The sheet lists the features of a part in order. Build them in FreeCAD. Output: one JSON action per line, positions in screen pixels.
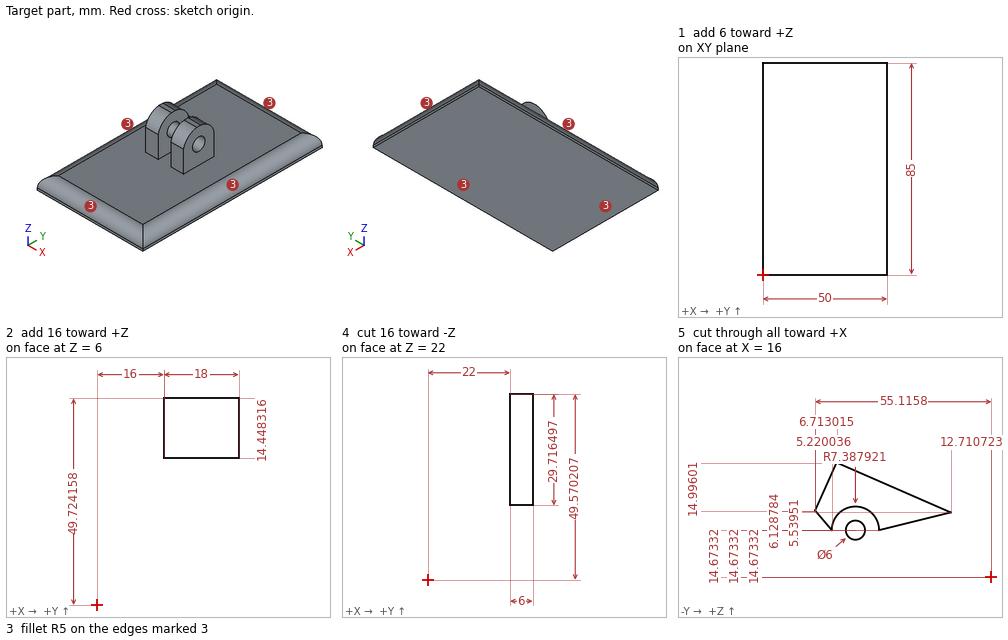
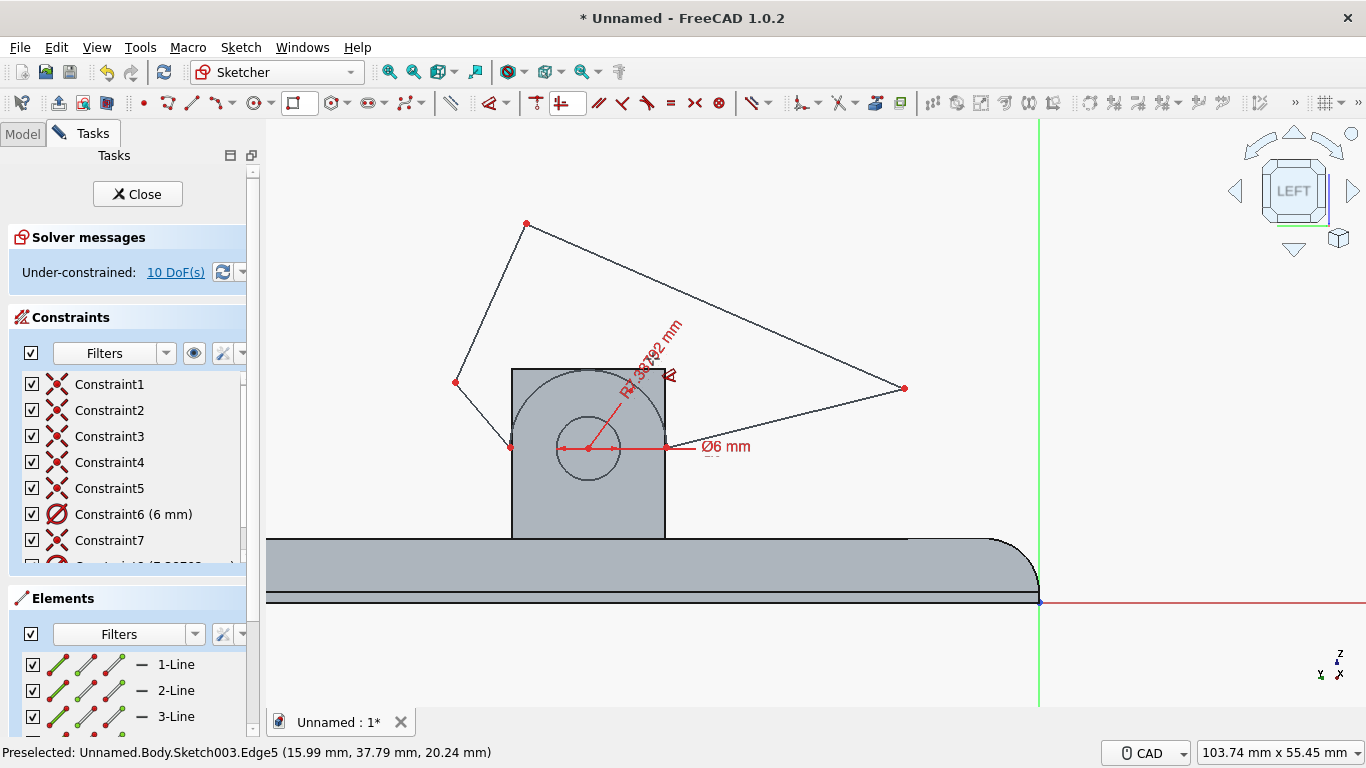
{"action": "left_click", "coordinate": [455, 383]}
{"action": "left_click", "coordinate": [747, 637]}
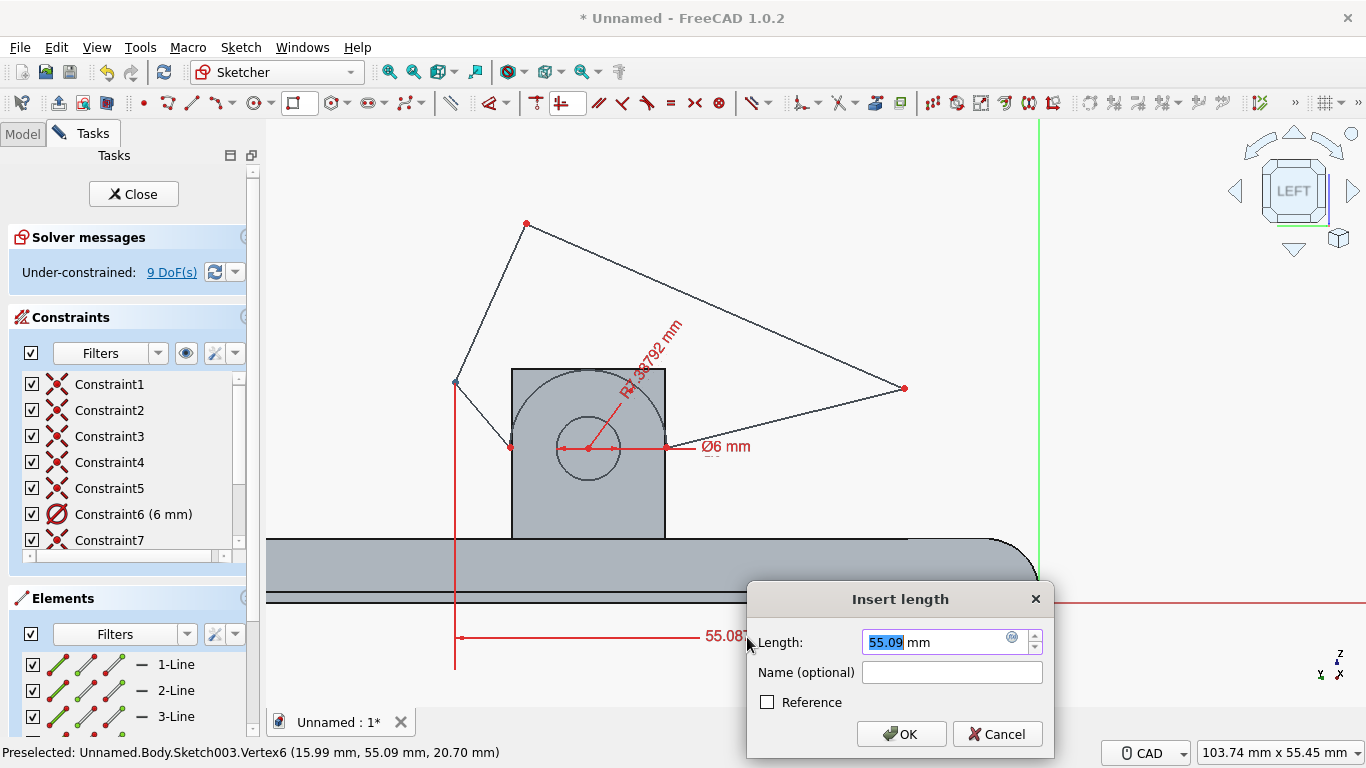
{"action": "type", "text": "55.1158"}
{"action": "key", "text": "Return"}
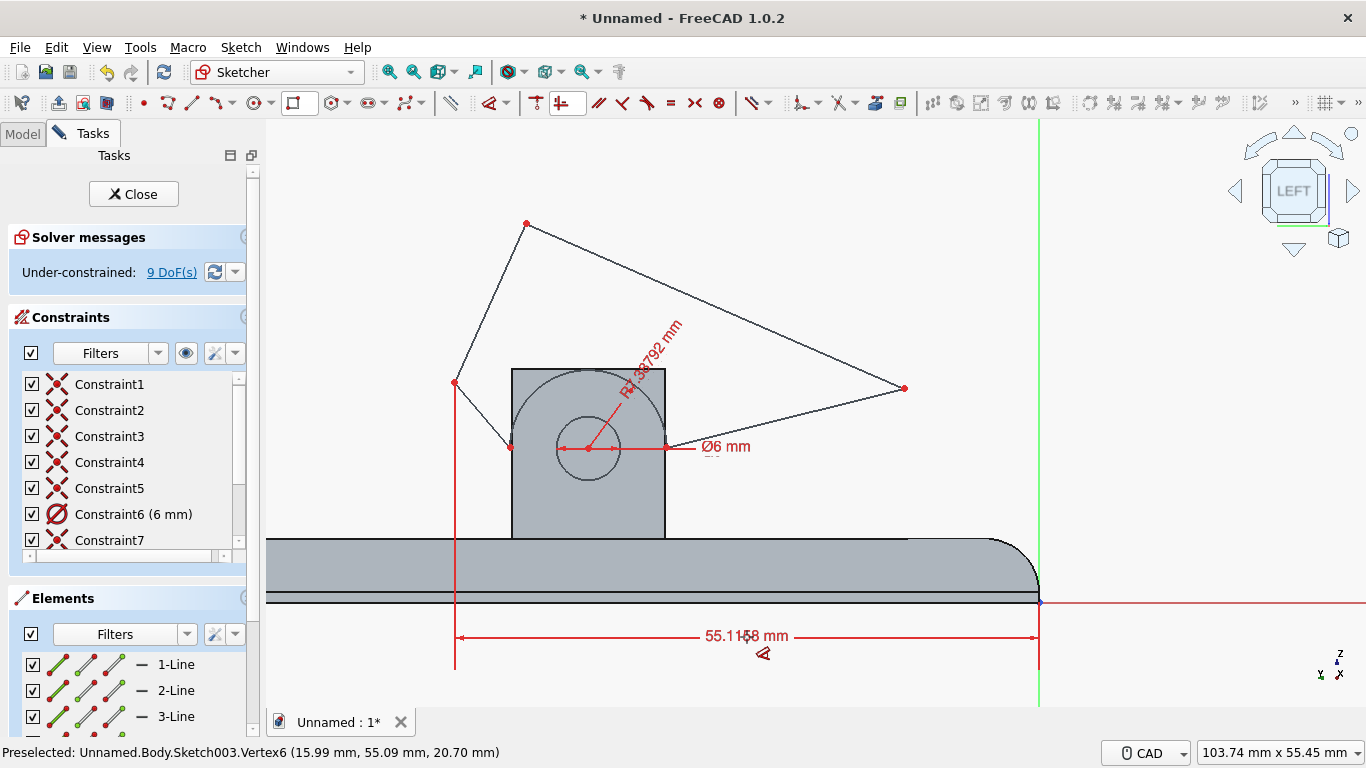
{"action": "left_click", "coordinate": [738, 430]}
{"action": "left_click", "coordinate": [938, 419]}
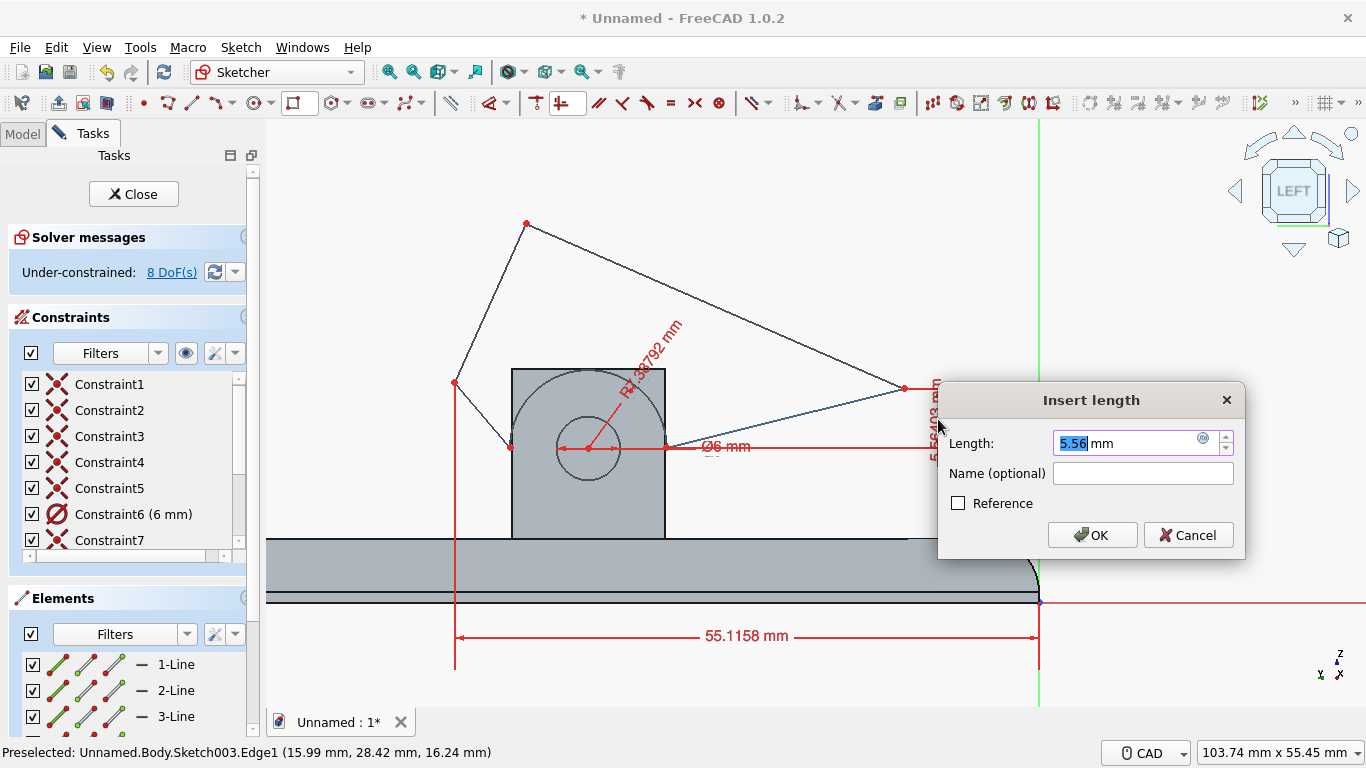
{"action": "type", "text": "5.53951"}
{"action": "key", "text": "Return"}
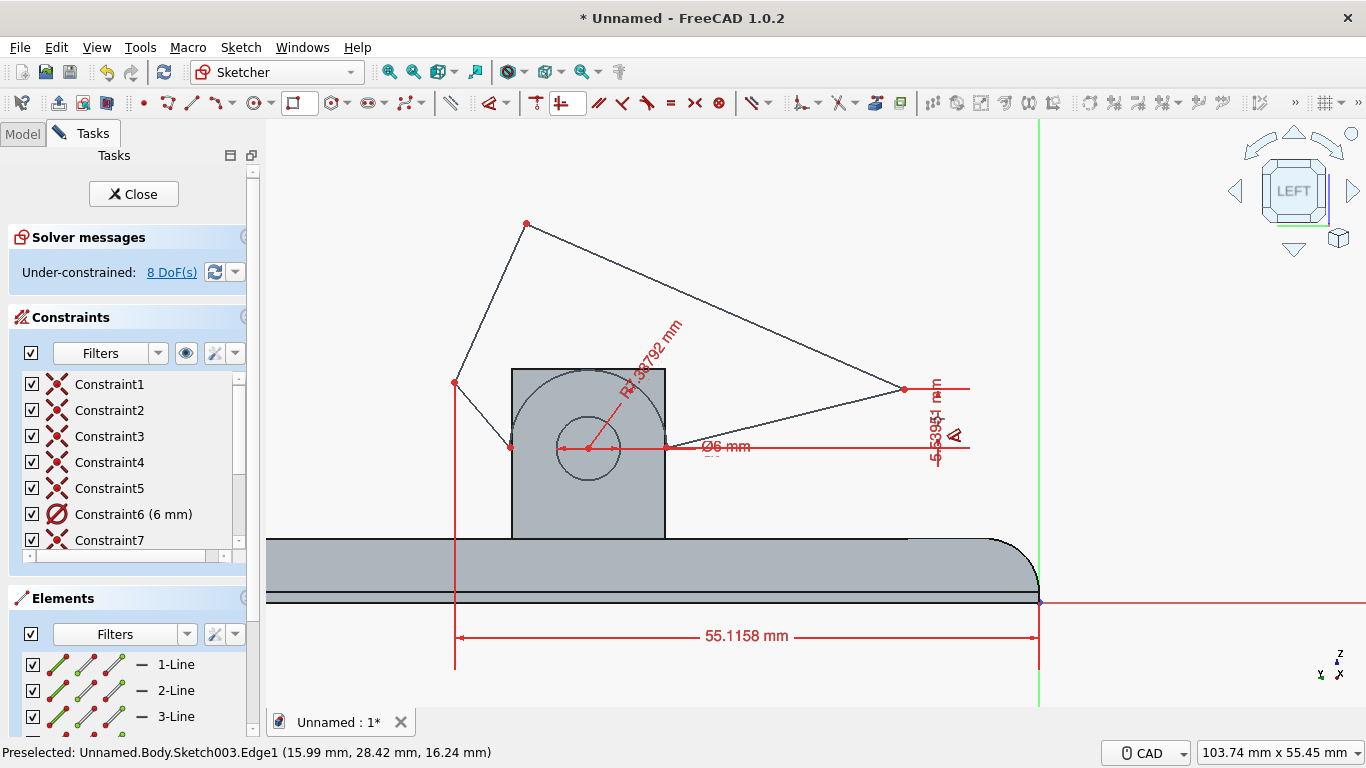
{"action": "left_click", "coordinate": [588, 449]}
{"action": "left_click", "coordinate": [1073, 526]}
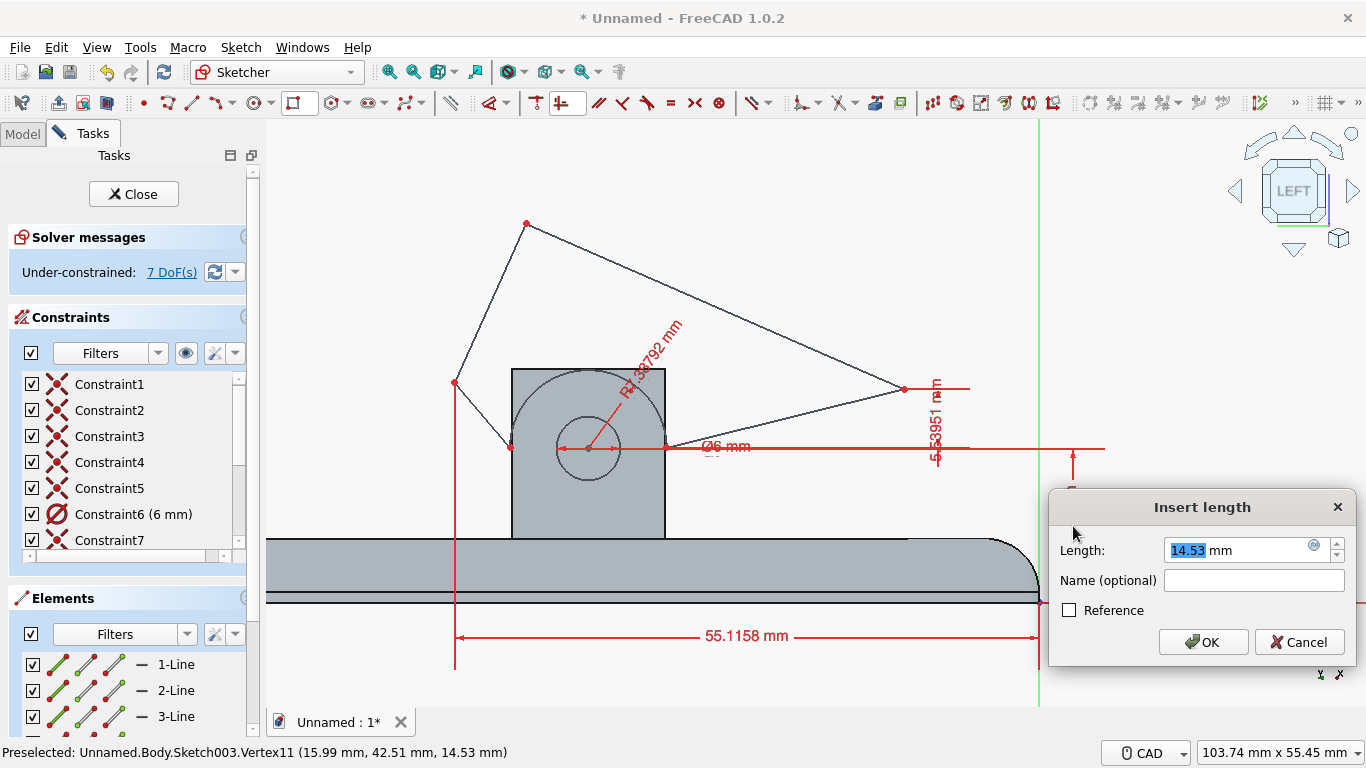
{"action": "type", "text": "14.67332"}
{"action": "key", "text": "Return"}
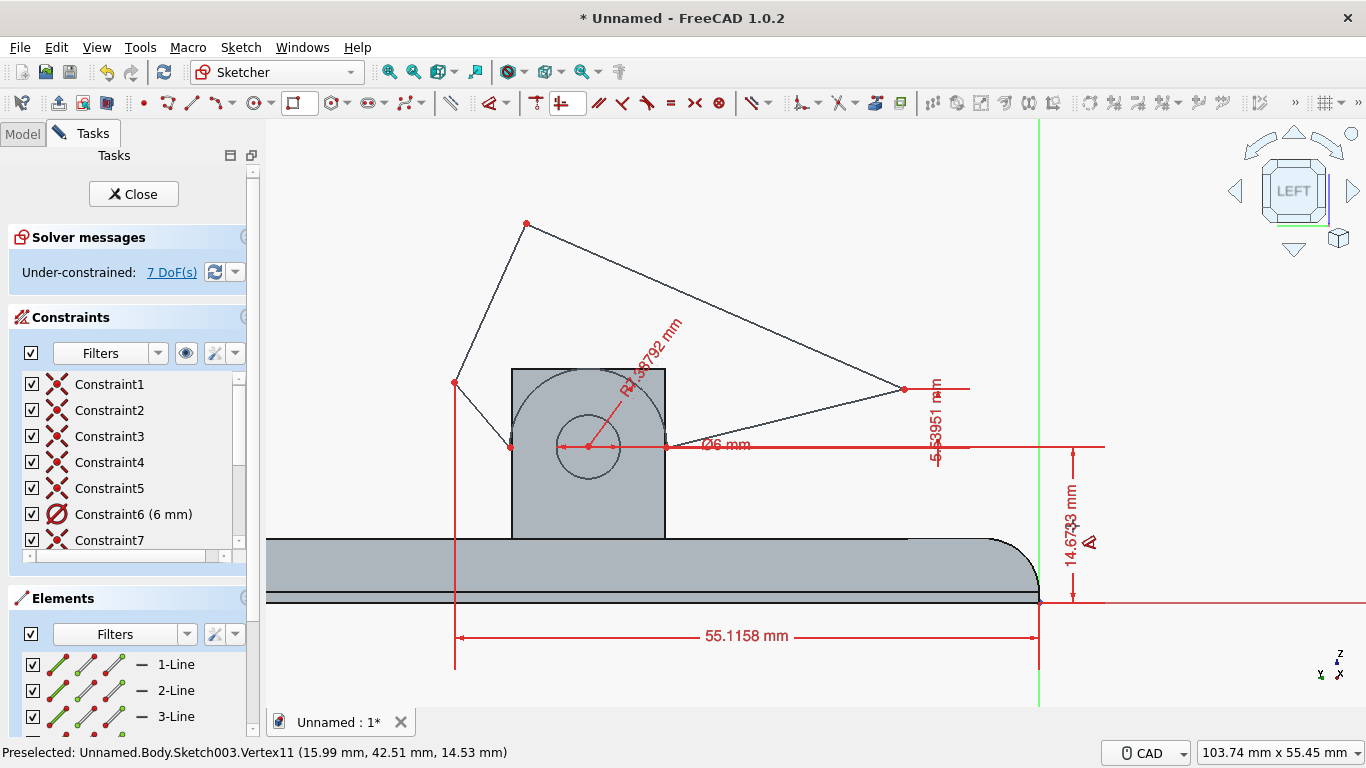
{"action": "left_click", "coordinate": [667, 448]}
{"action": "left_click", "coordinate": [1073, 490]}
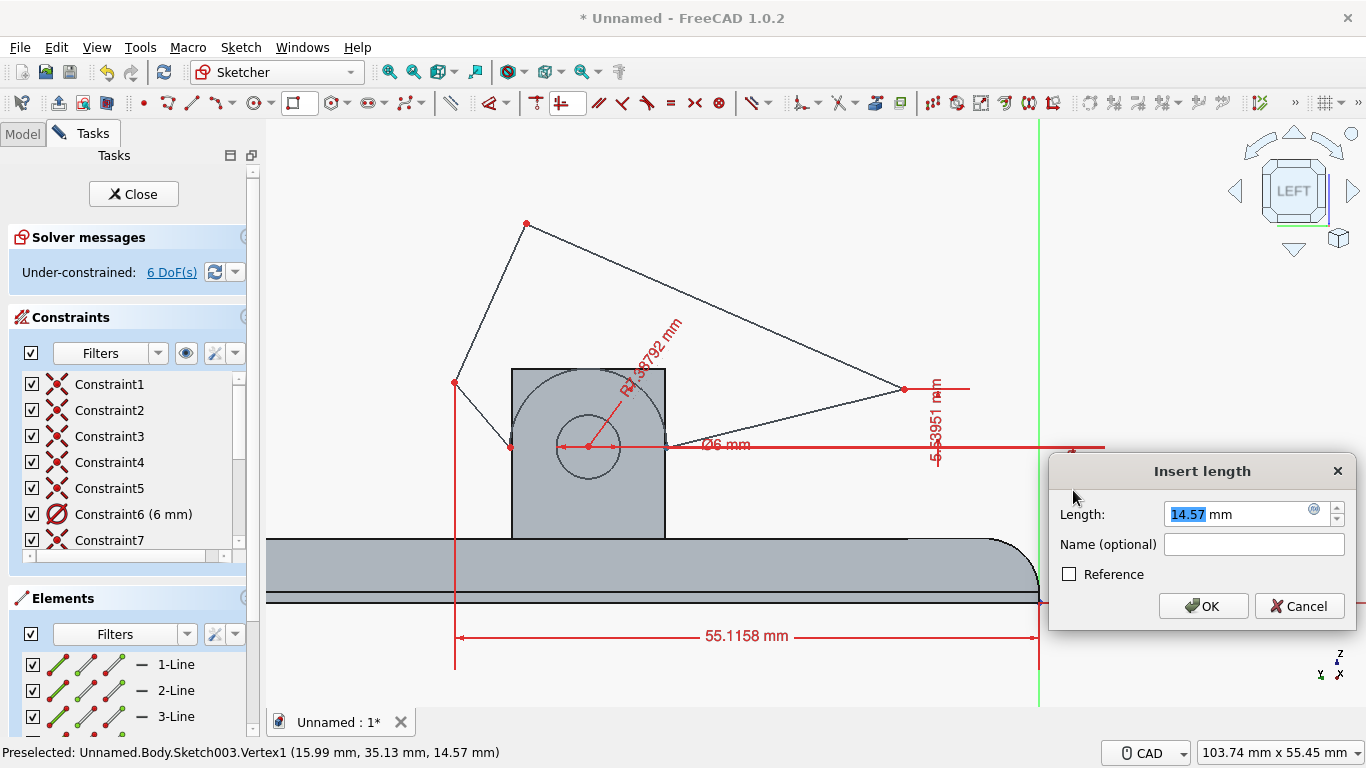
{"action": "type", "text": "14.67332"}
{"action": "key", "text": "Return"}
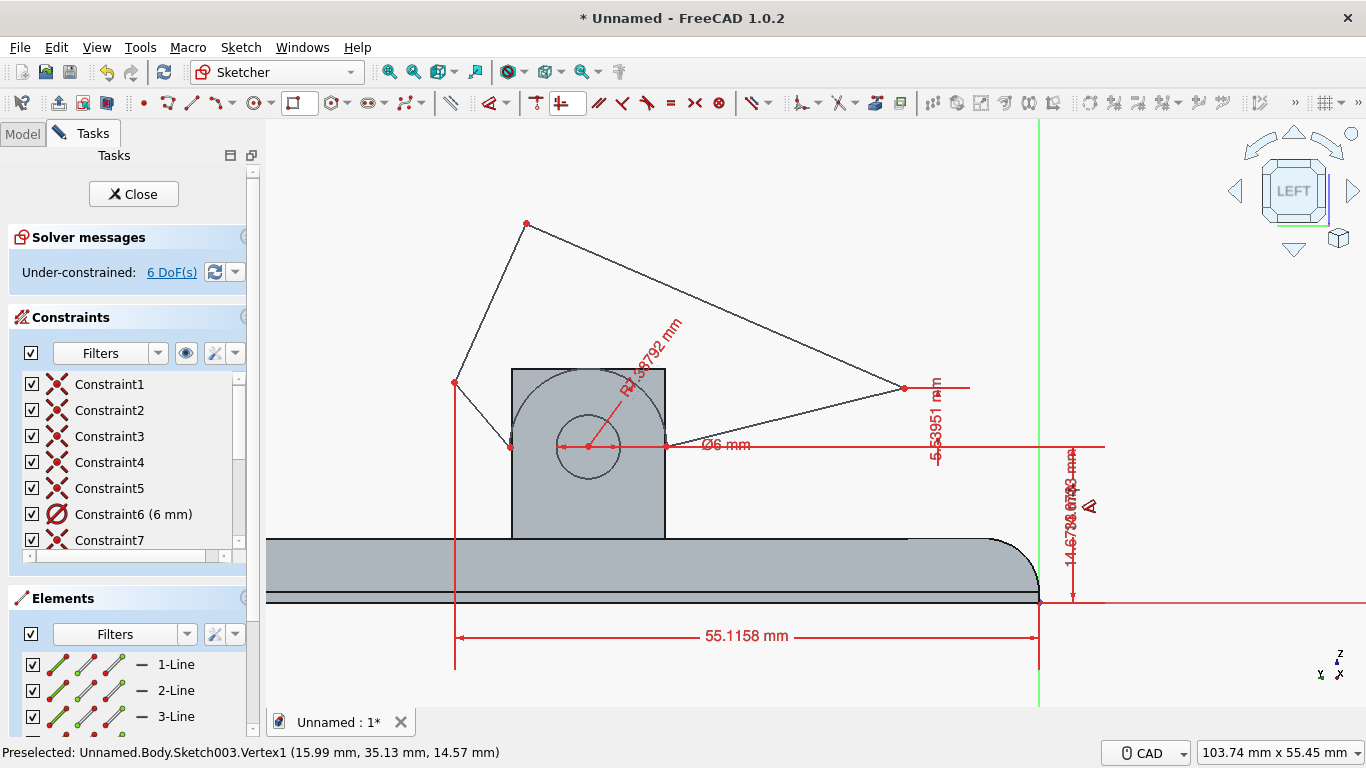
{"action": "left_click", "coordinate": [510, 448]}
{"action": "left_click", "coordinate": [1073, 561]}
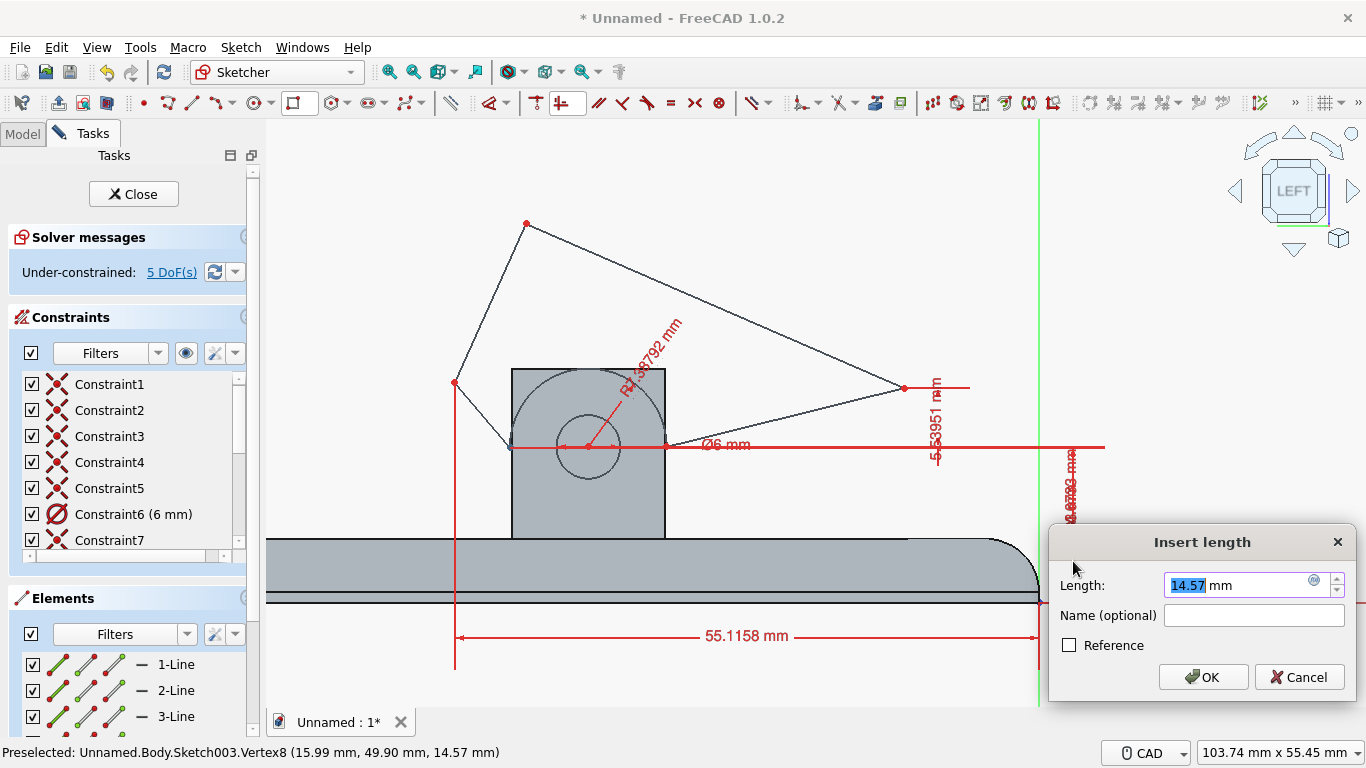
{"action": "type", "text": "14.67332"}
{"action": "key", "text": "Return"}